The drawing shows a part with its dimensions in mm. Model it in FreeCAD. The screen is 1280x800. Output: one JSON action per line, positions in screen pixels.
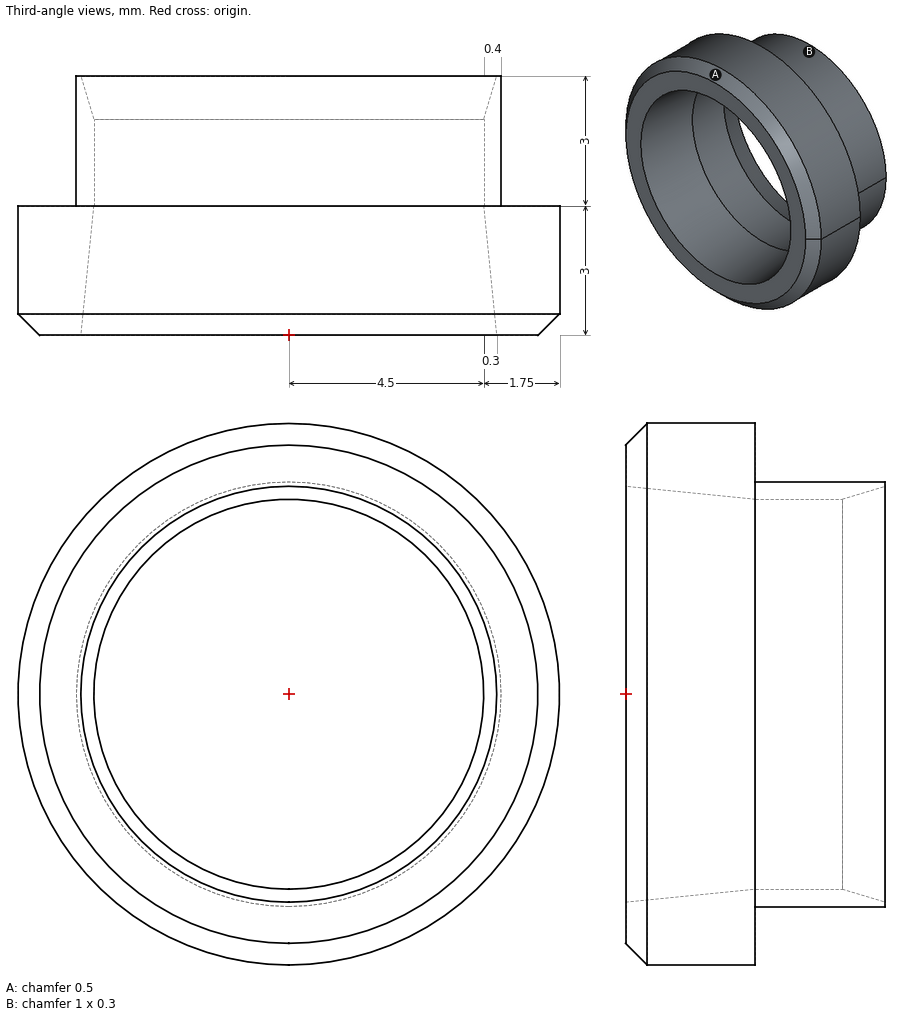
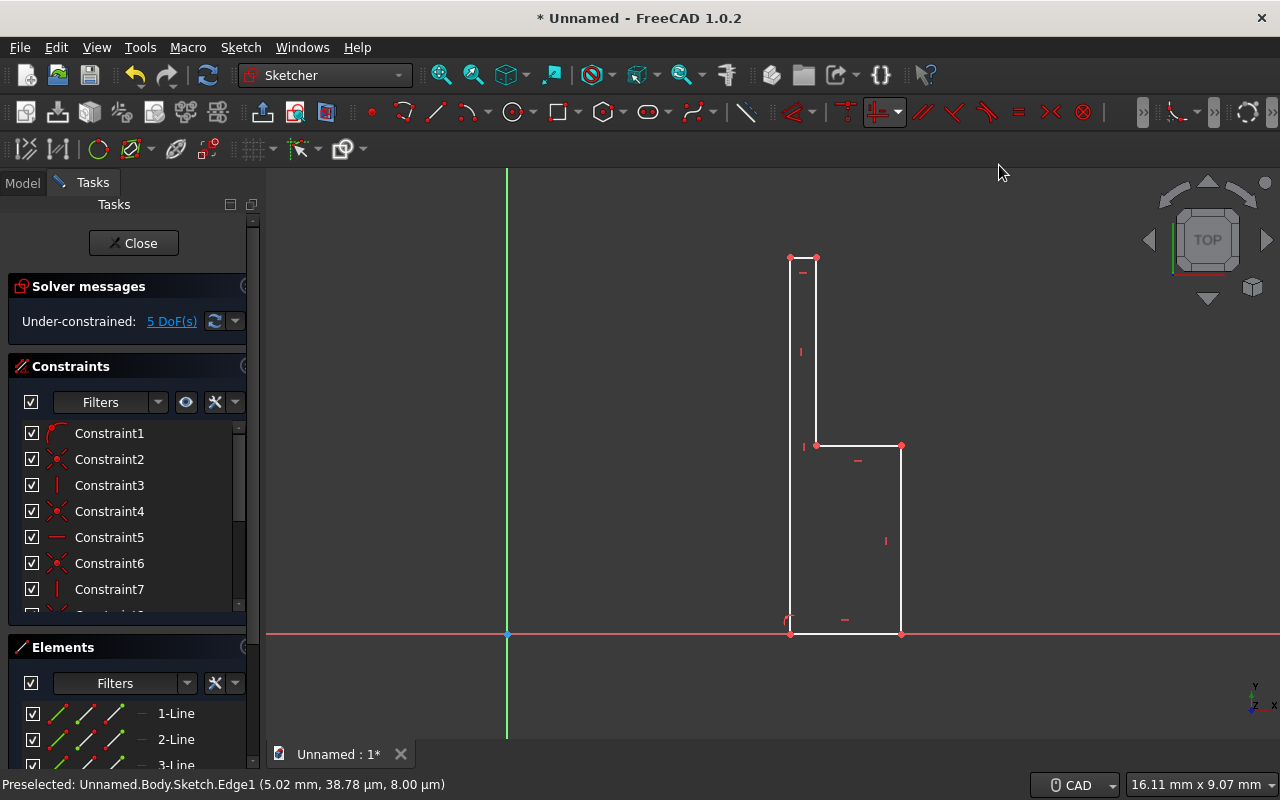
{"action": "key", "text": "d"}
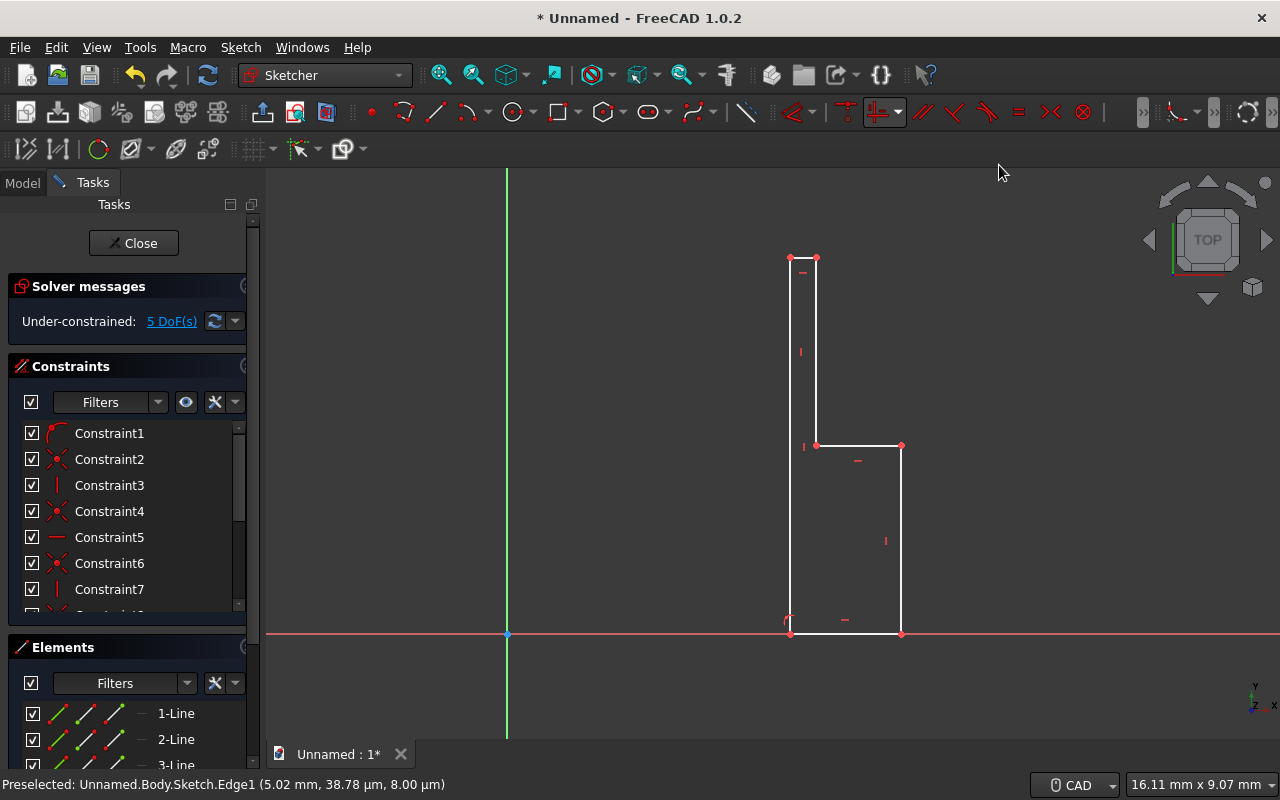
{"action": "left_click", "coordinate": [901, 578]}
{"action": "left_click", "coordinate": [935, 540]}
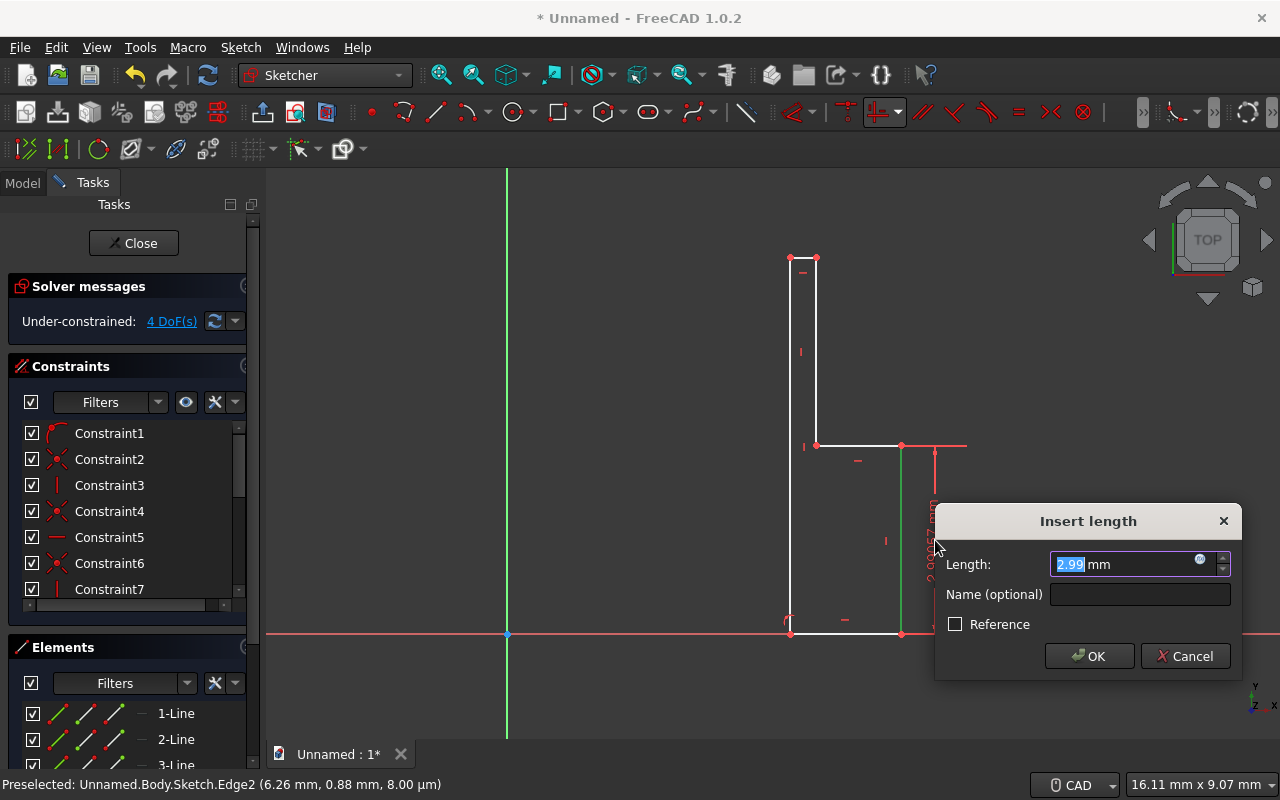
{"action": "type", "text": "3"}
{"action": "key", "text": "Return"}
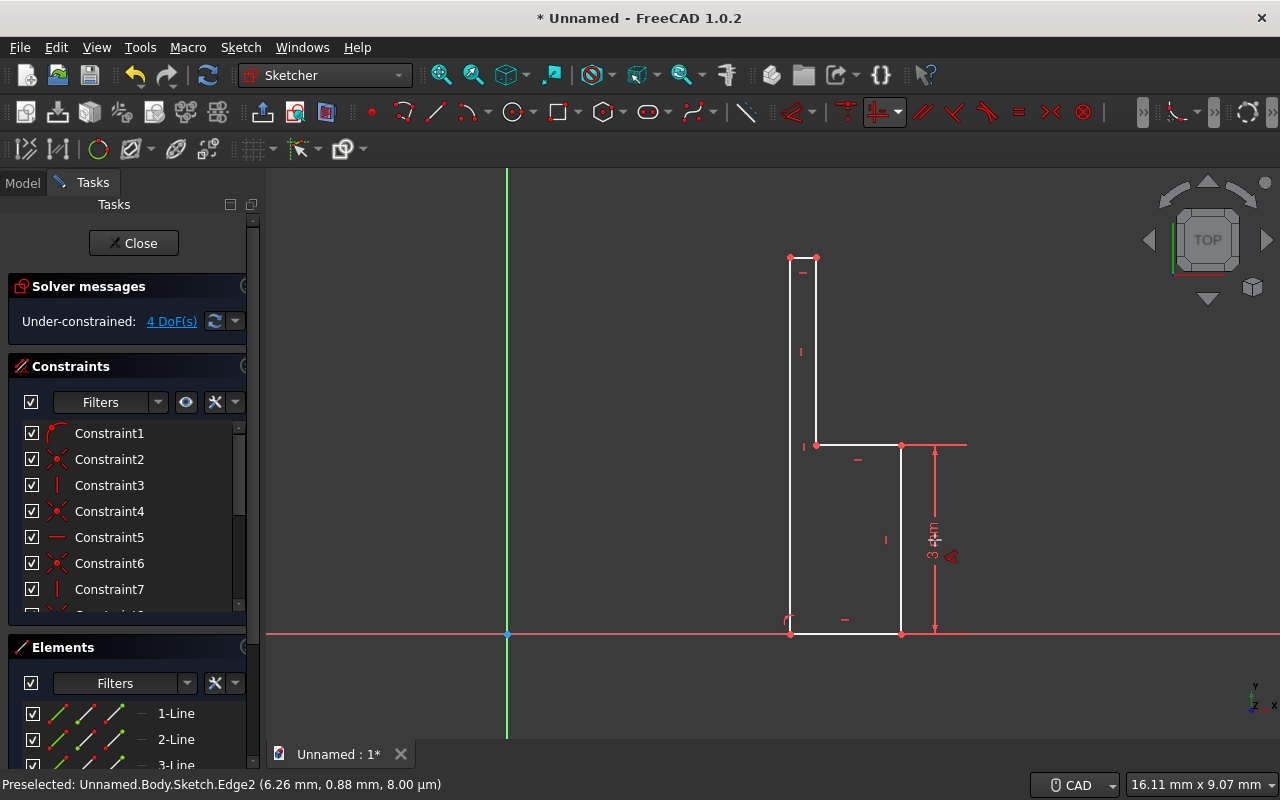
{"action": "left_click", "coordinate": [816, 389]}
{"action": "left_click", "coordinate": [850, 352]}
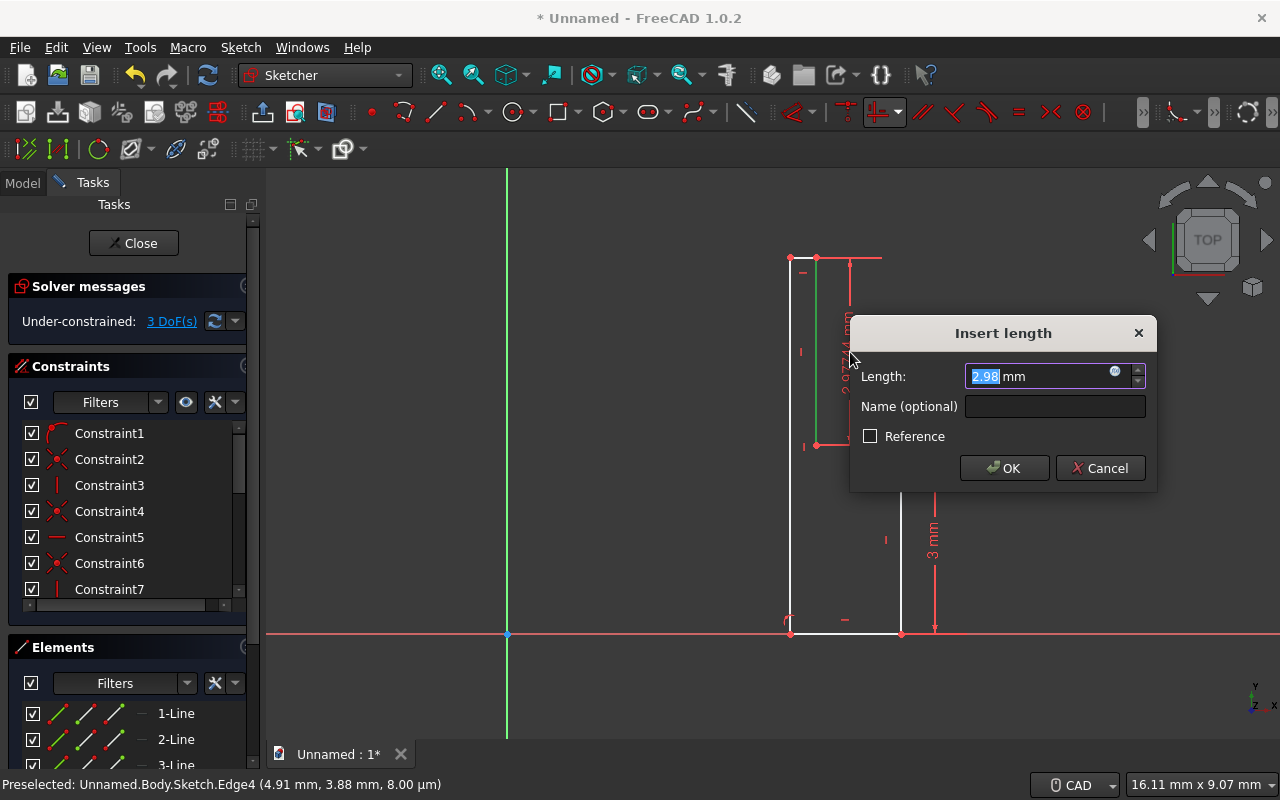
{"action": "type", "text": "3"}
{"action": "key", "text": "Return"}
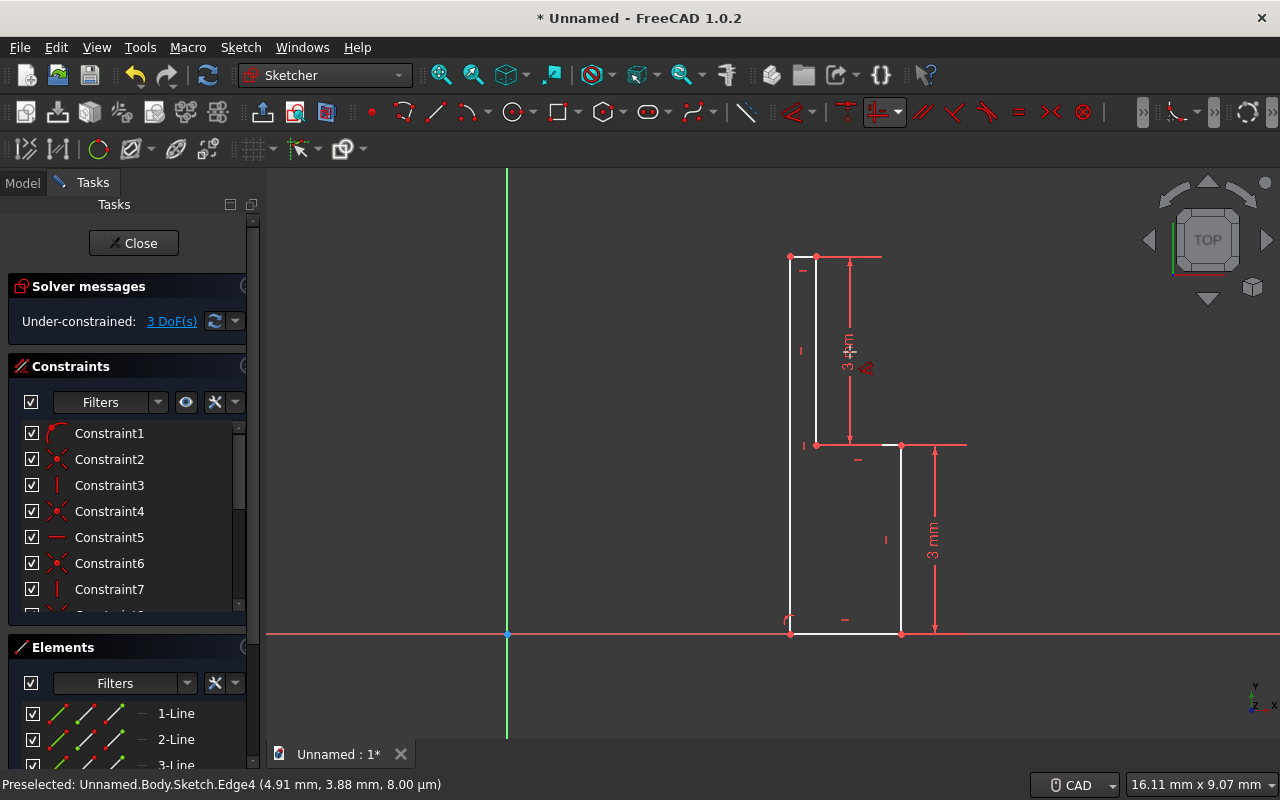
{"action": "scroll", "coordinate": [806, 257], "scroll_direction": "up", "scroll_amount": 3}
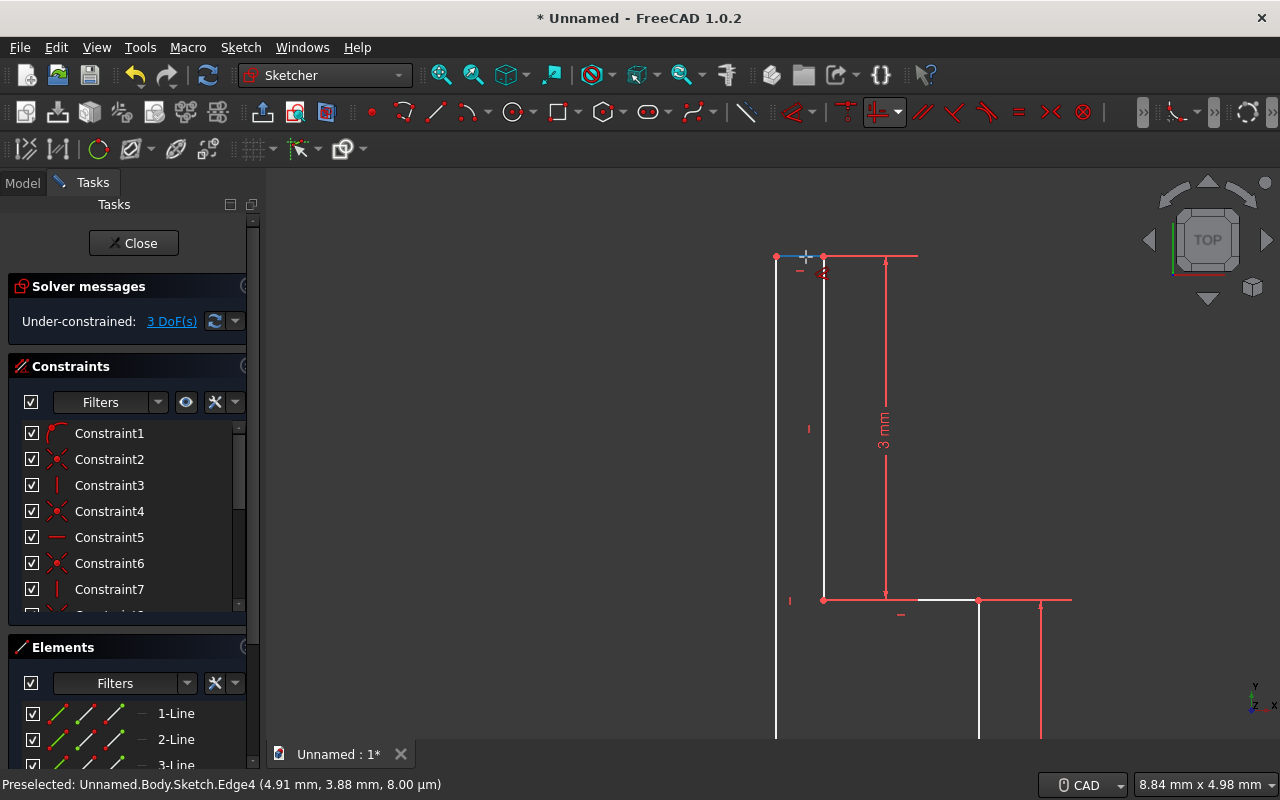
{"action": "left_click", "coordinate": [805, 256]}
{"action": "left_click", "coordinate": [800, 222]}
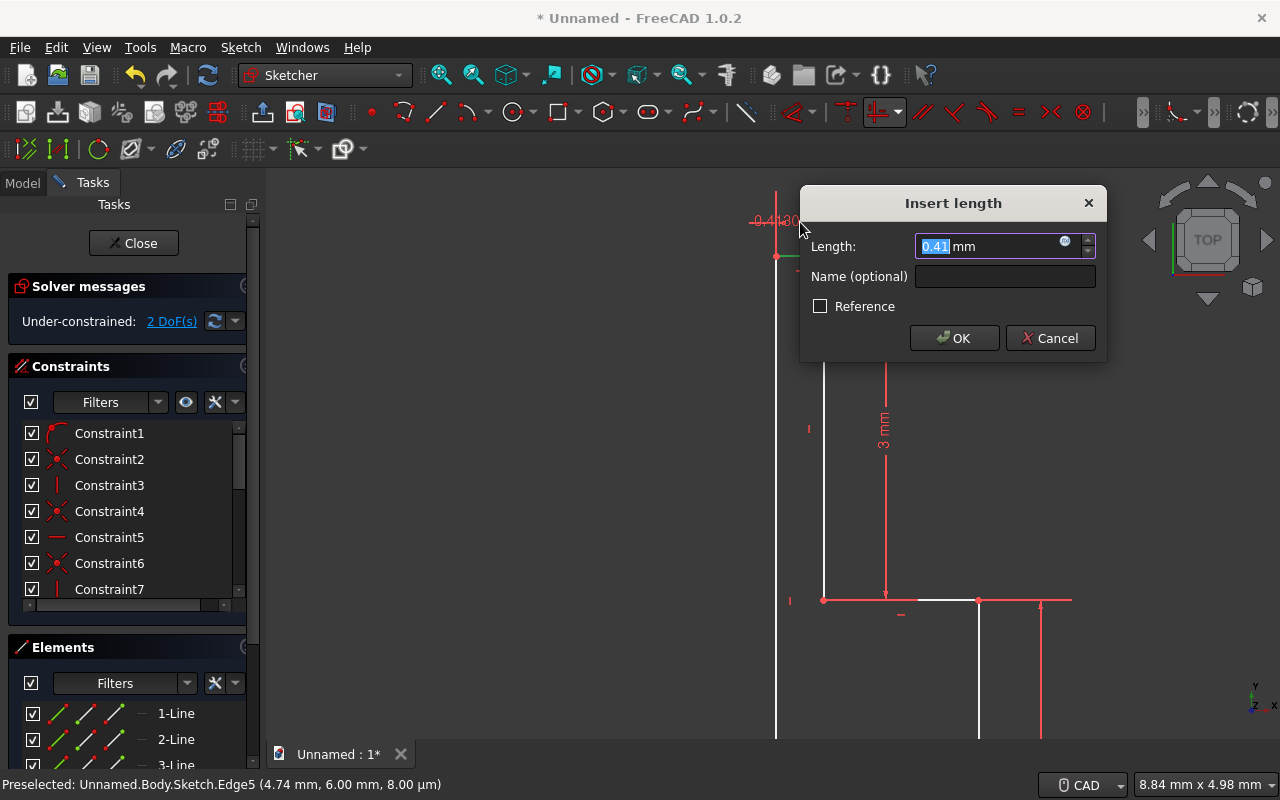
{"action": "type", "text": "0.4"}
{"action": "key", "text": "Return"}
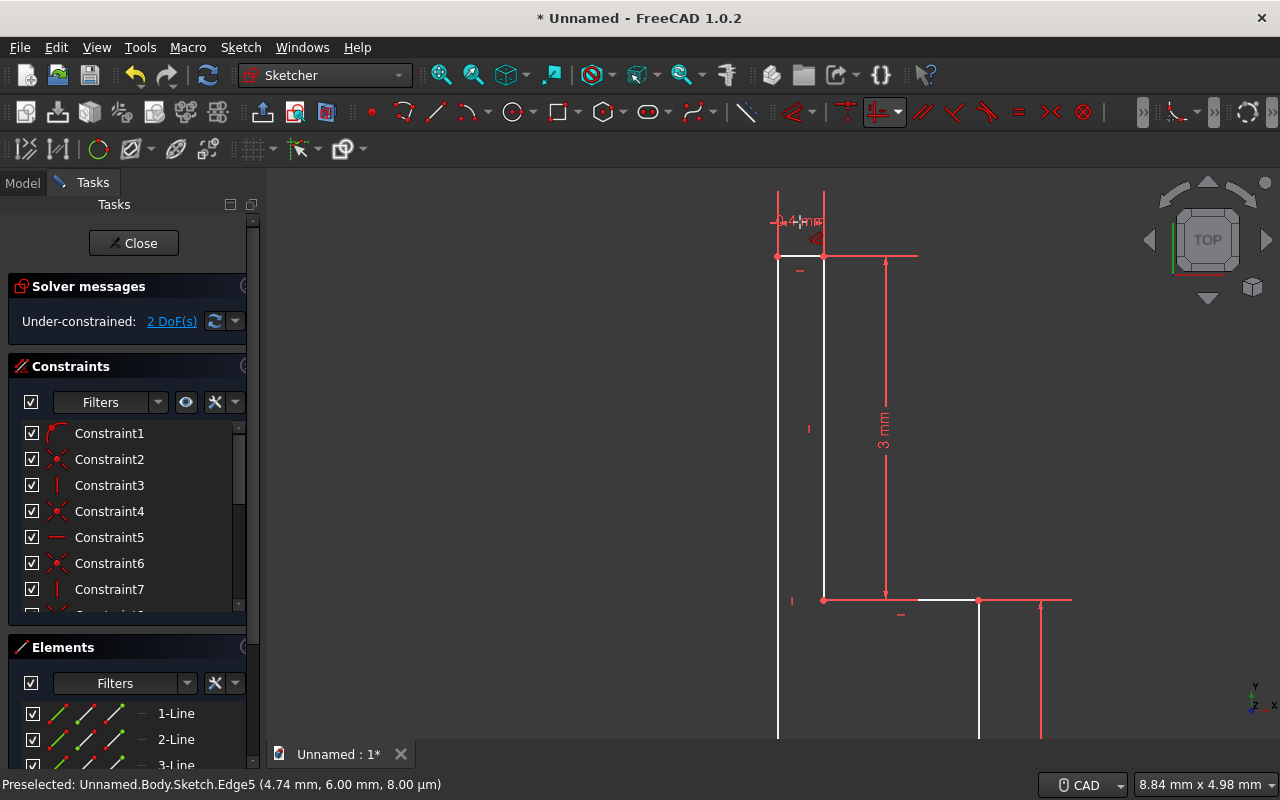
{"action": "scroll", "coordinate": [808, 275], "scroll_direction": "down", "scroll_amount": 3}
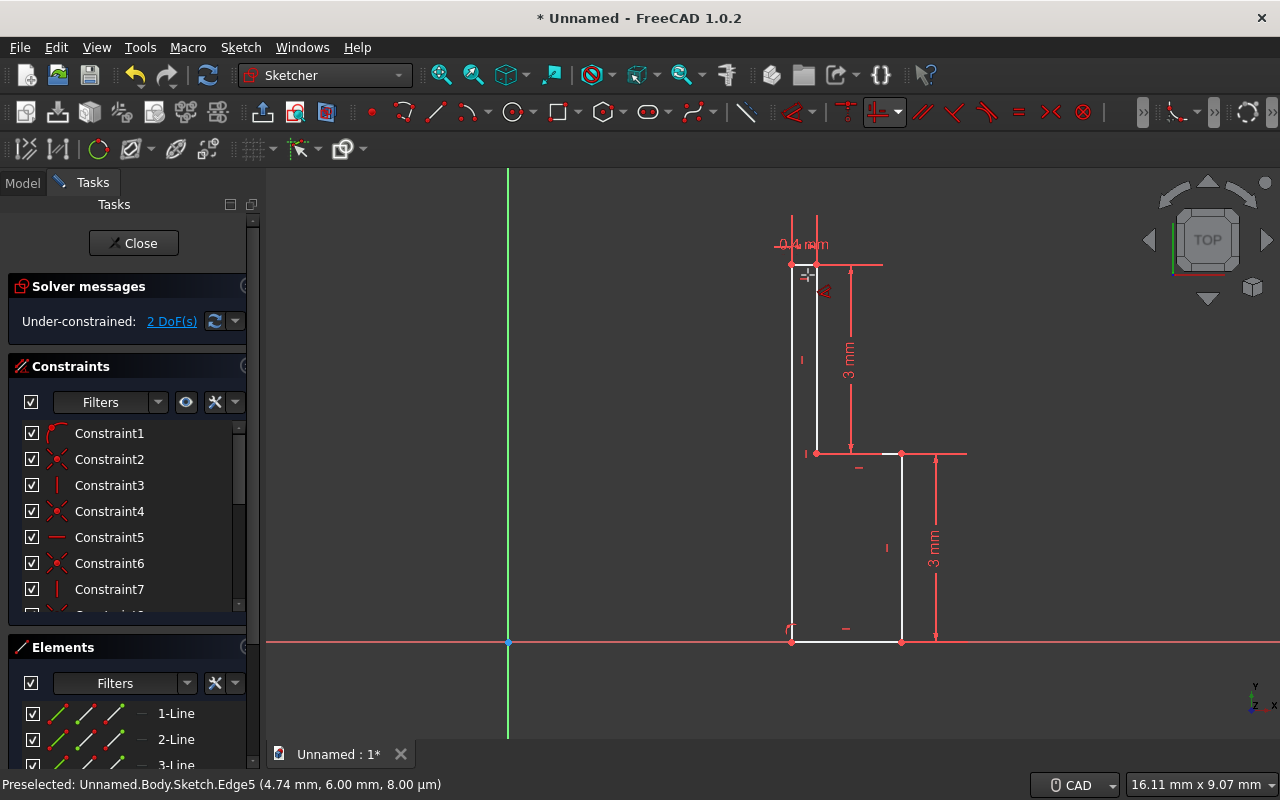
{"action": "left_click", "coordinate": [825, 642]}
{"action": "left_click", "coordinate": [847, 676]}